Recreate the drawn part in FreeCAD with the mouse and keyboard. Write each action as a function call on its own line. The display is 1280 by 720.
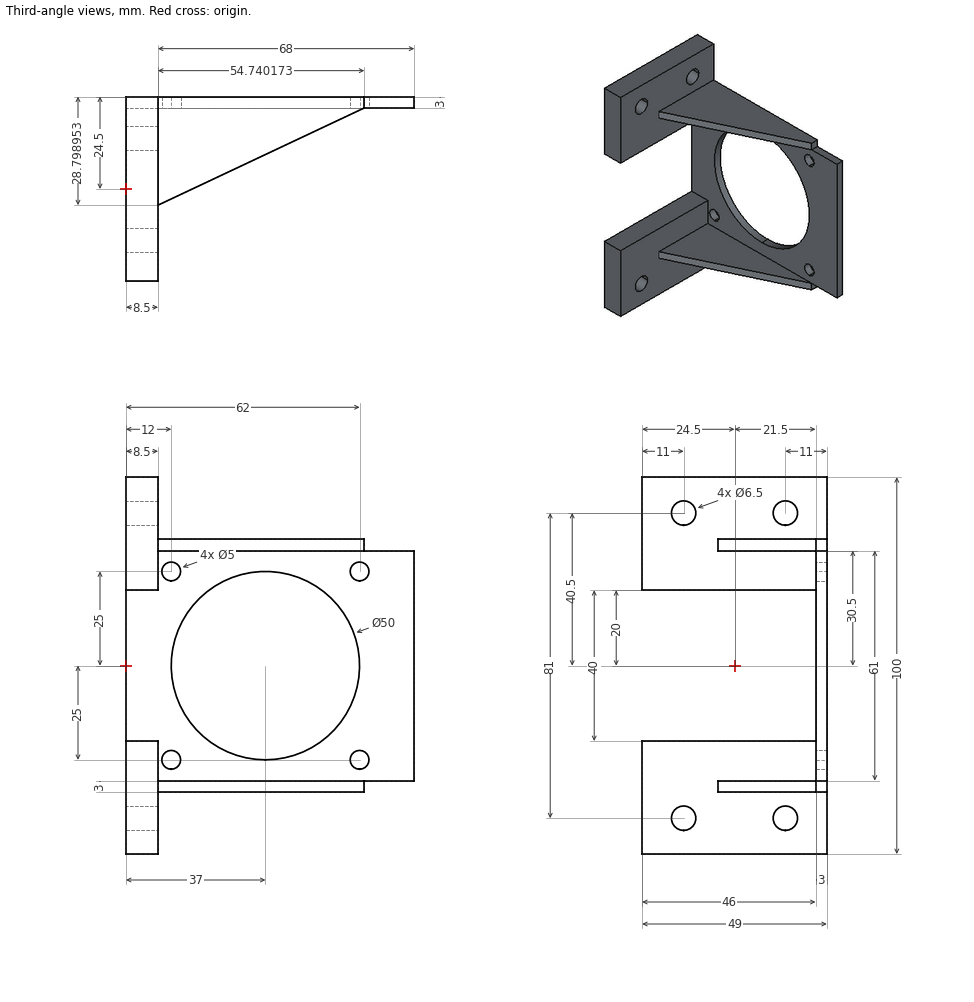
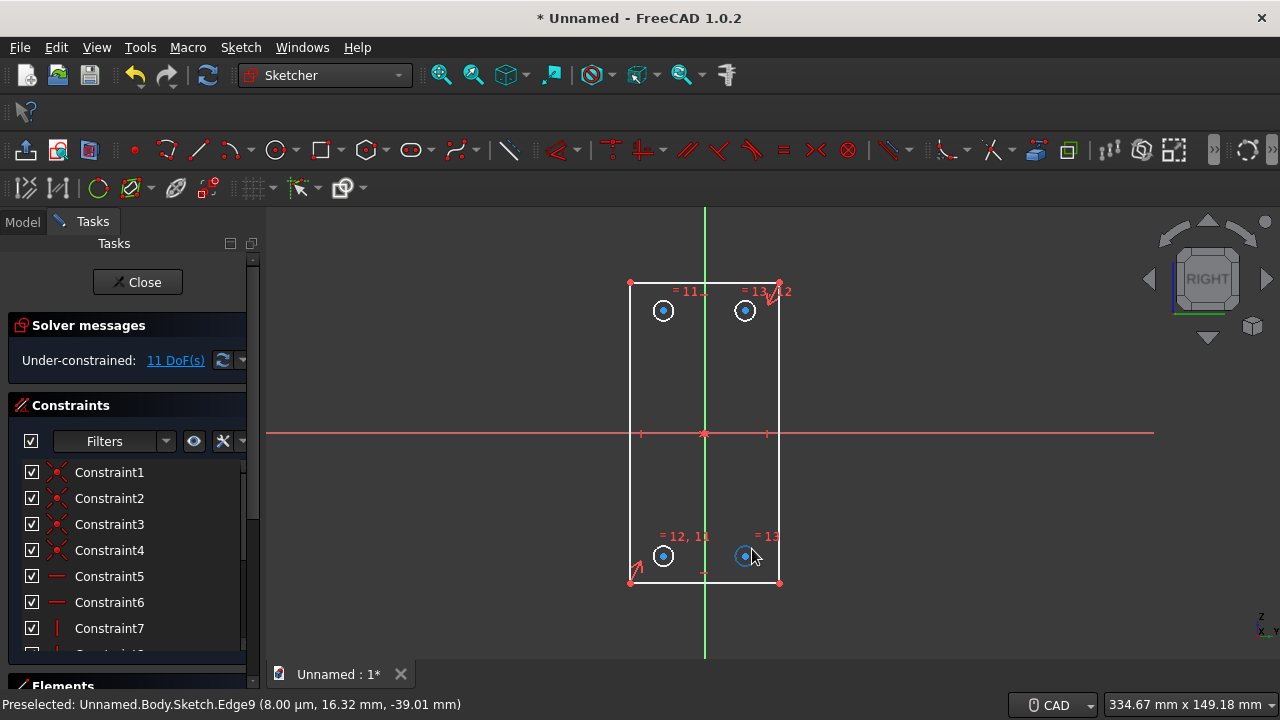
click(664, 311)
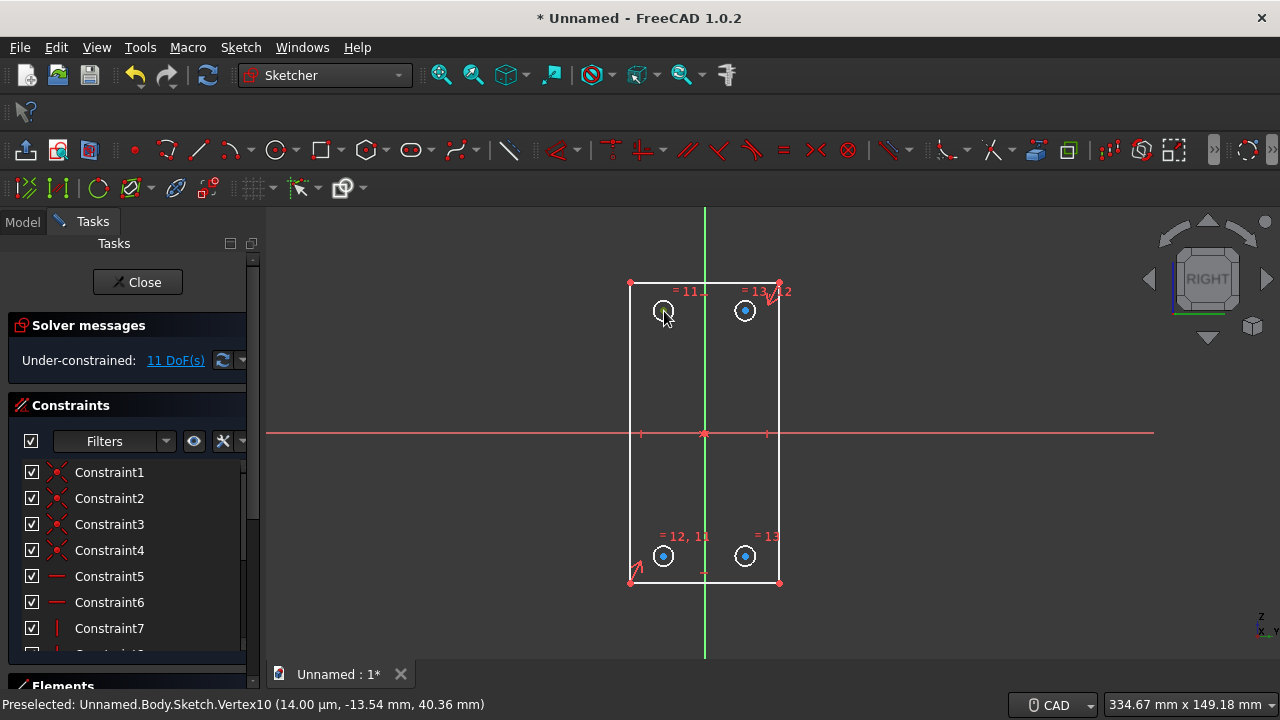
click(664, 556)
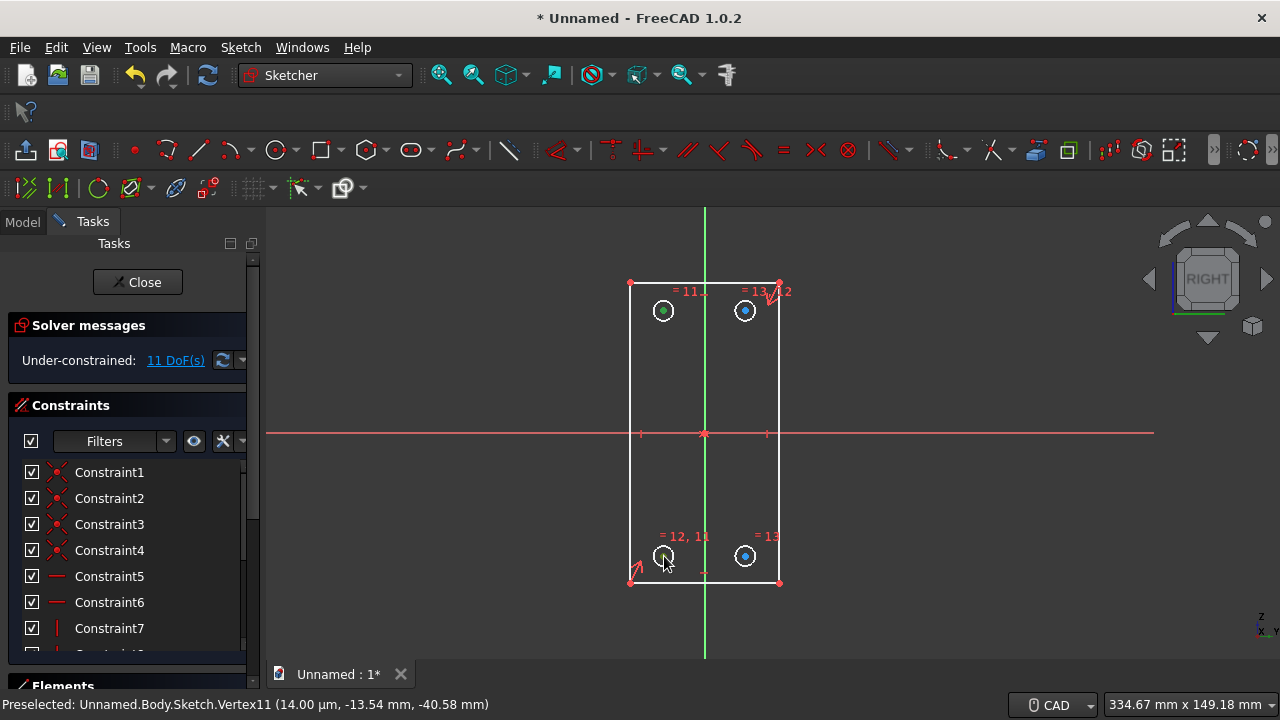
key(v)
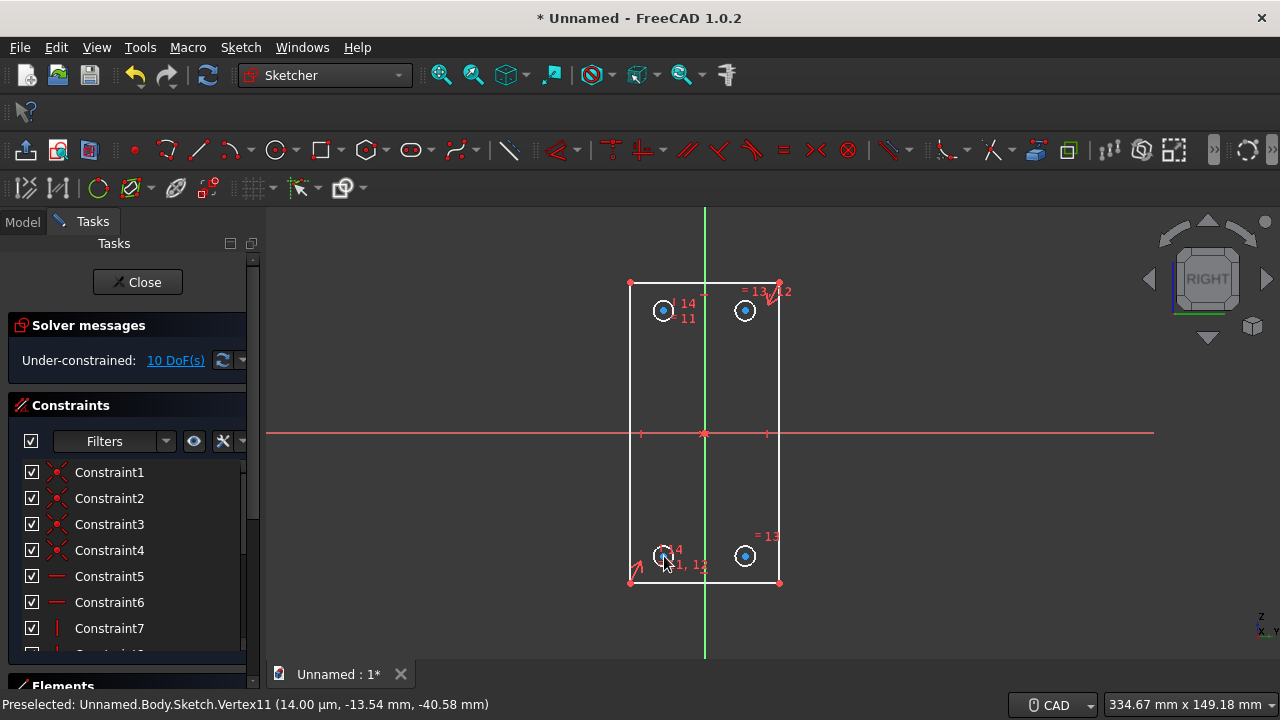
click(664, 311)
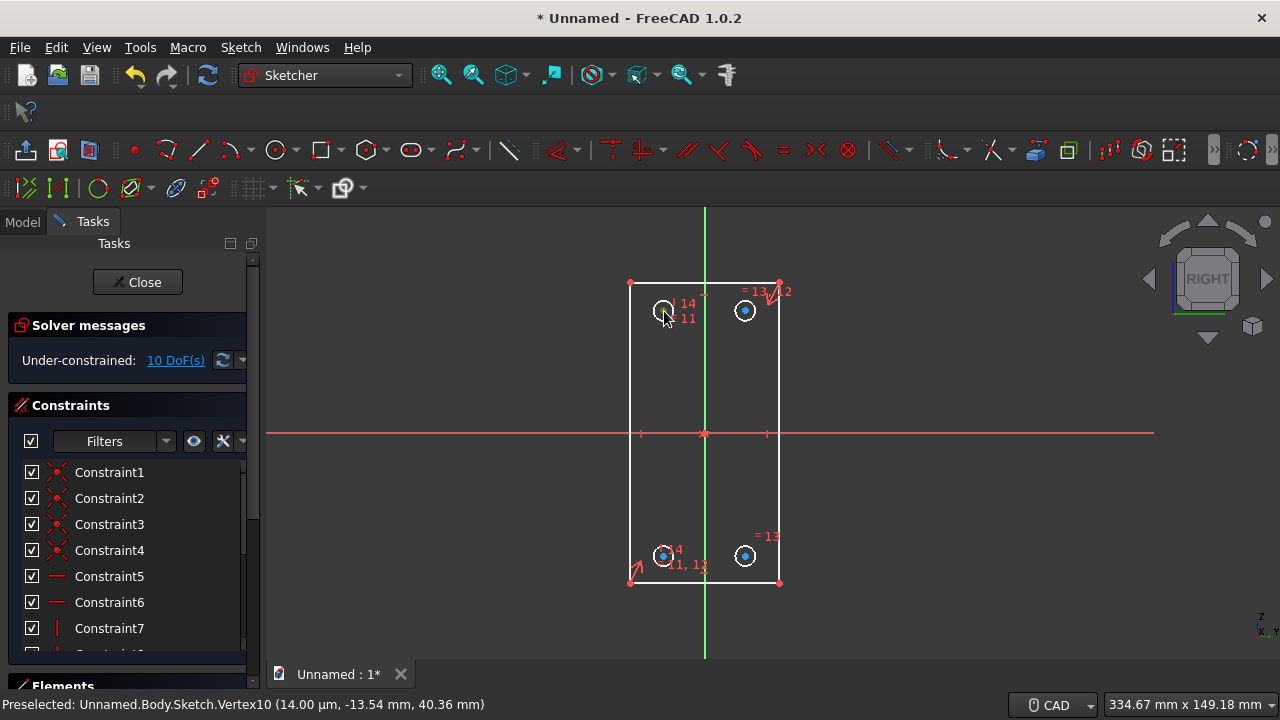
click(745, 311)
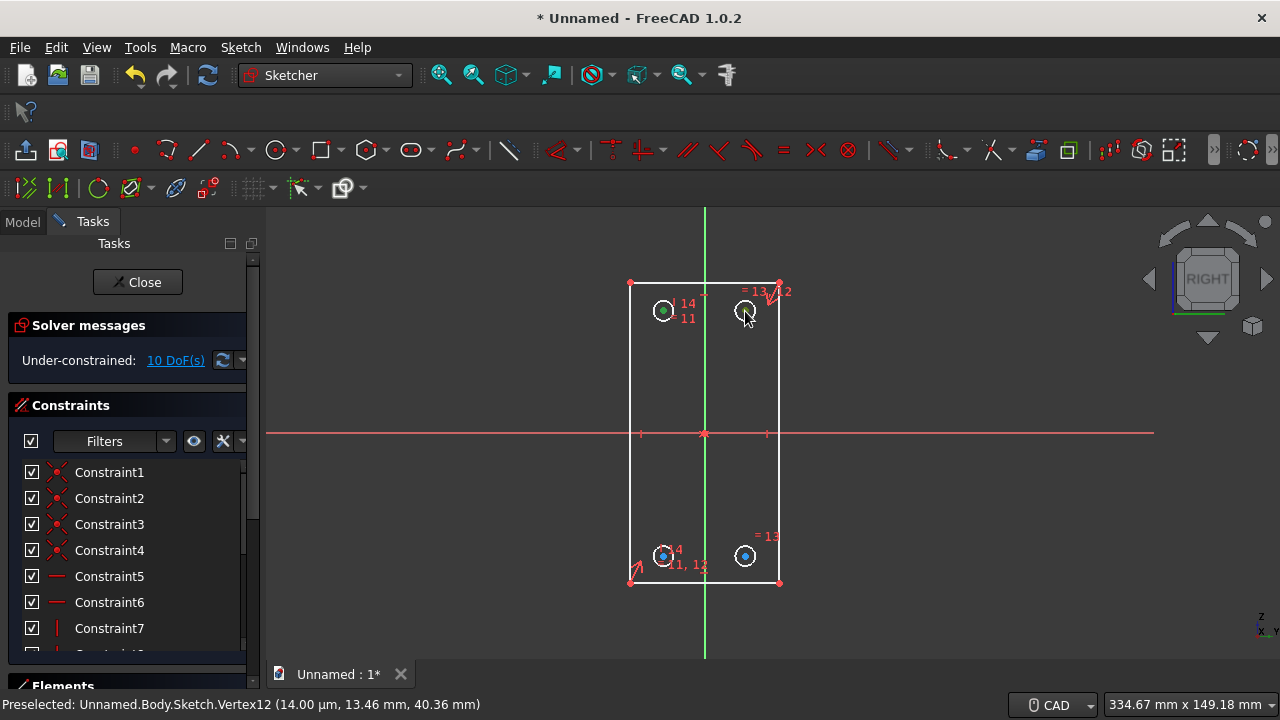
key(h)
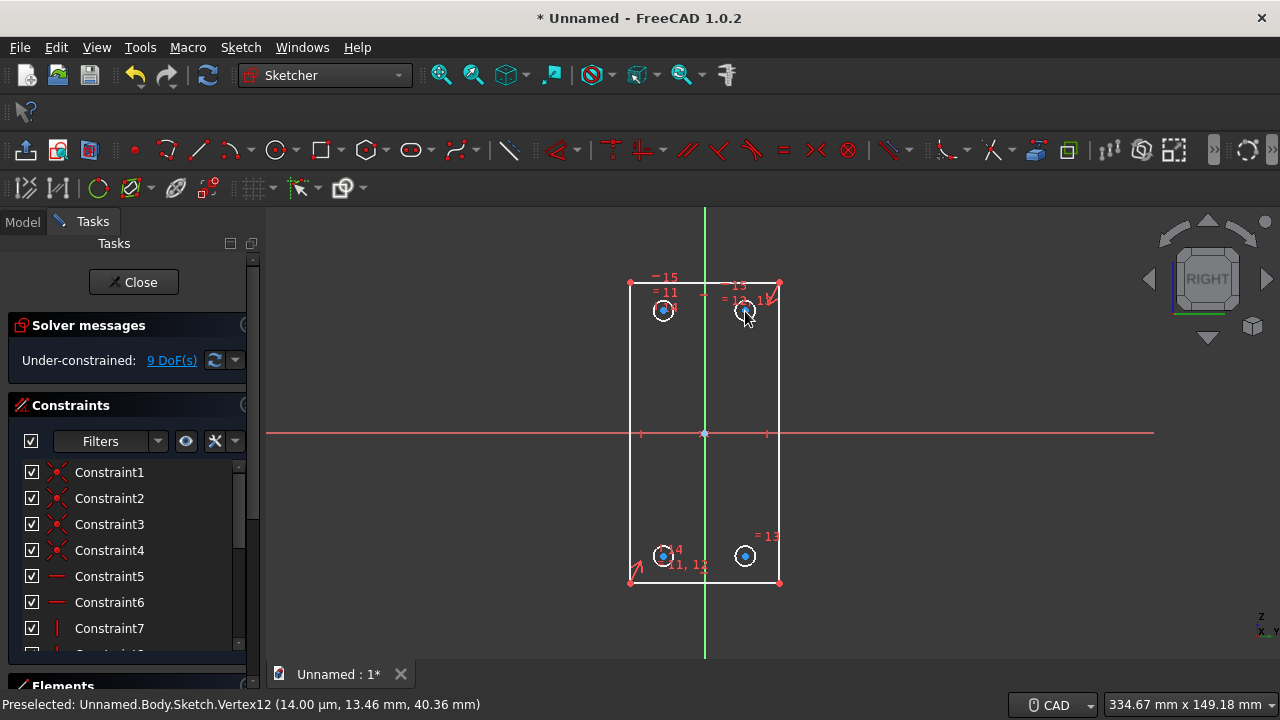
click(745, 311)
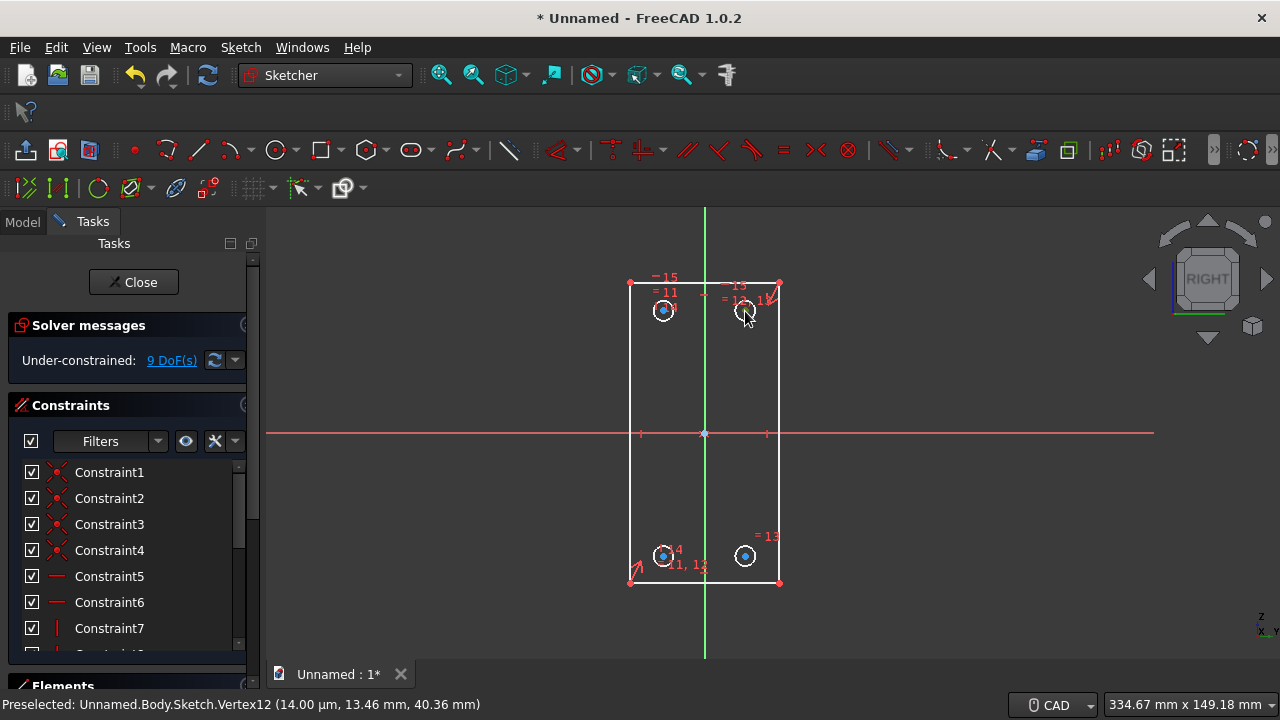
click(745, 556)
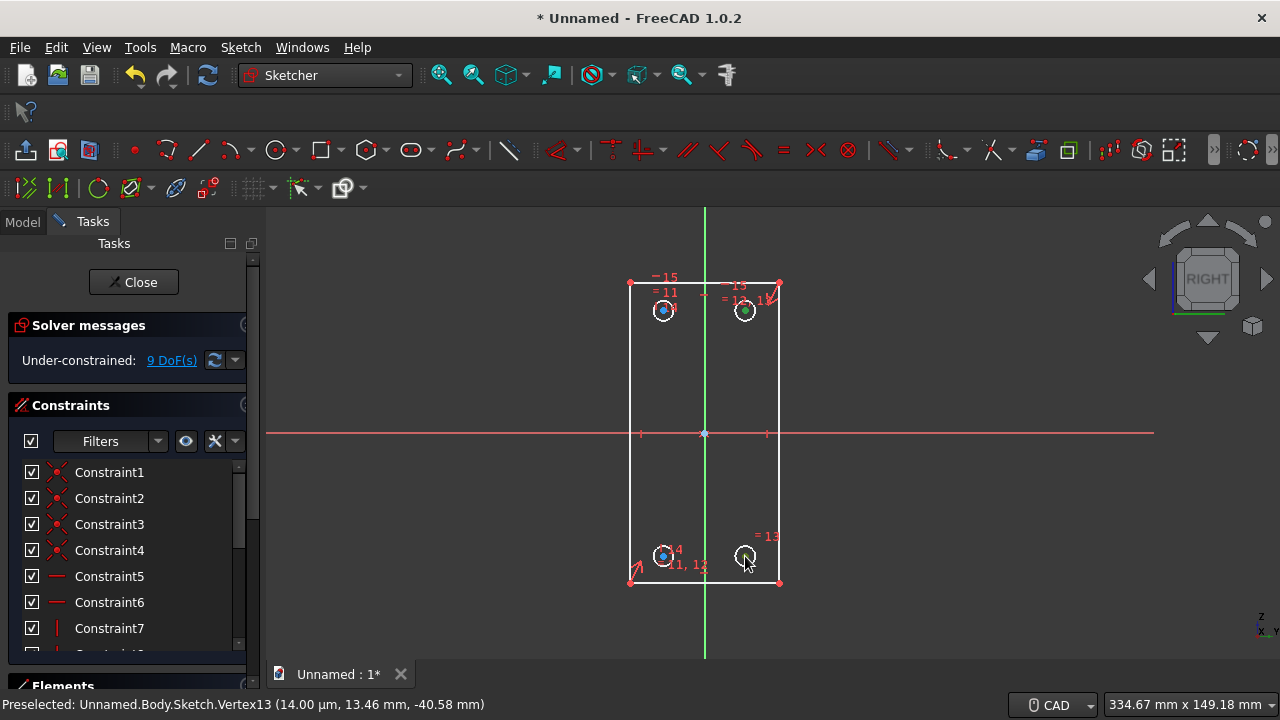
click(666, 150)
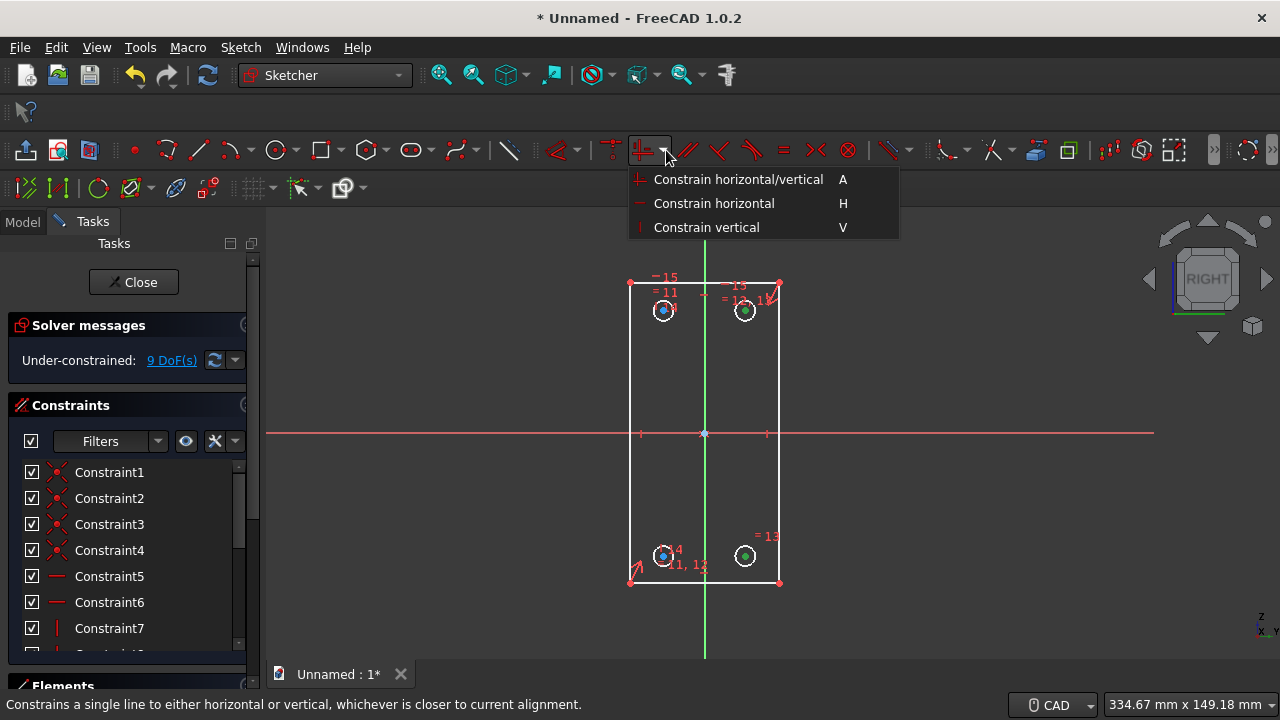
click(764, 227)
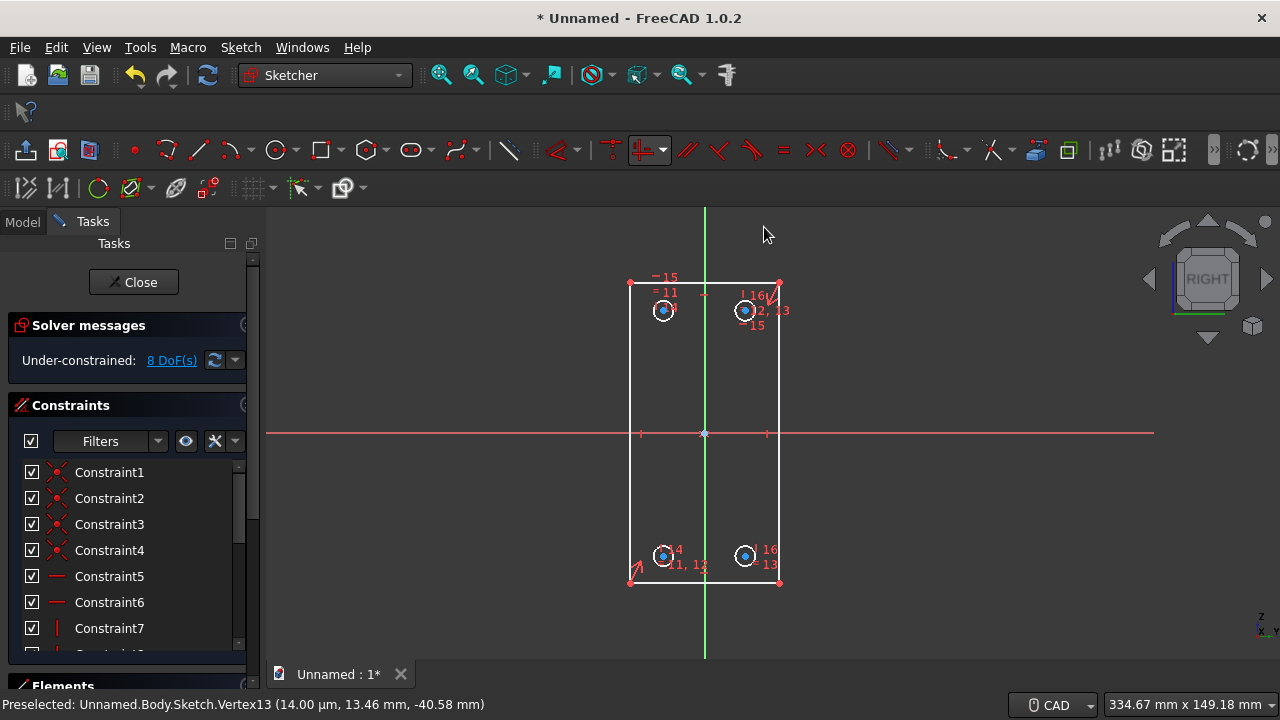
scroll(664, 556, up, 4)